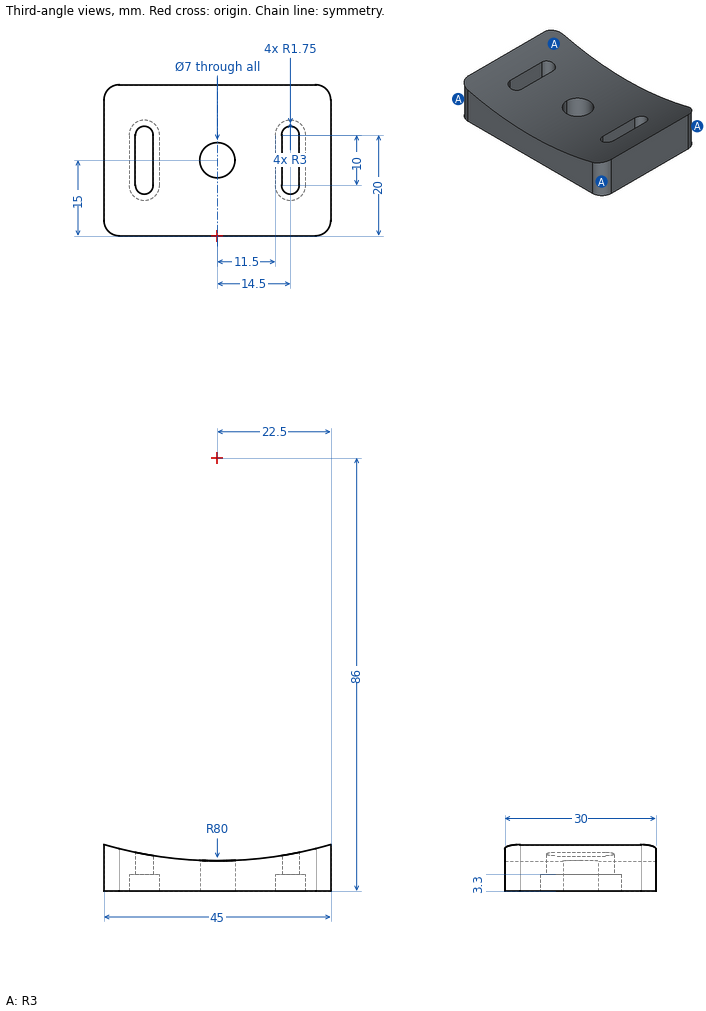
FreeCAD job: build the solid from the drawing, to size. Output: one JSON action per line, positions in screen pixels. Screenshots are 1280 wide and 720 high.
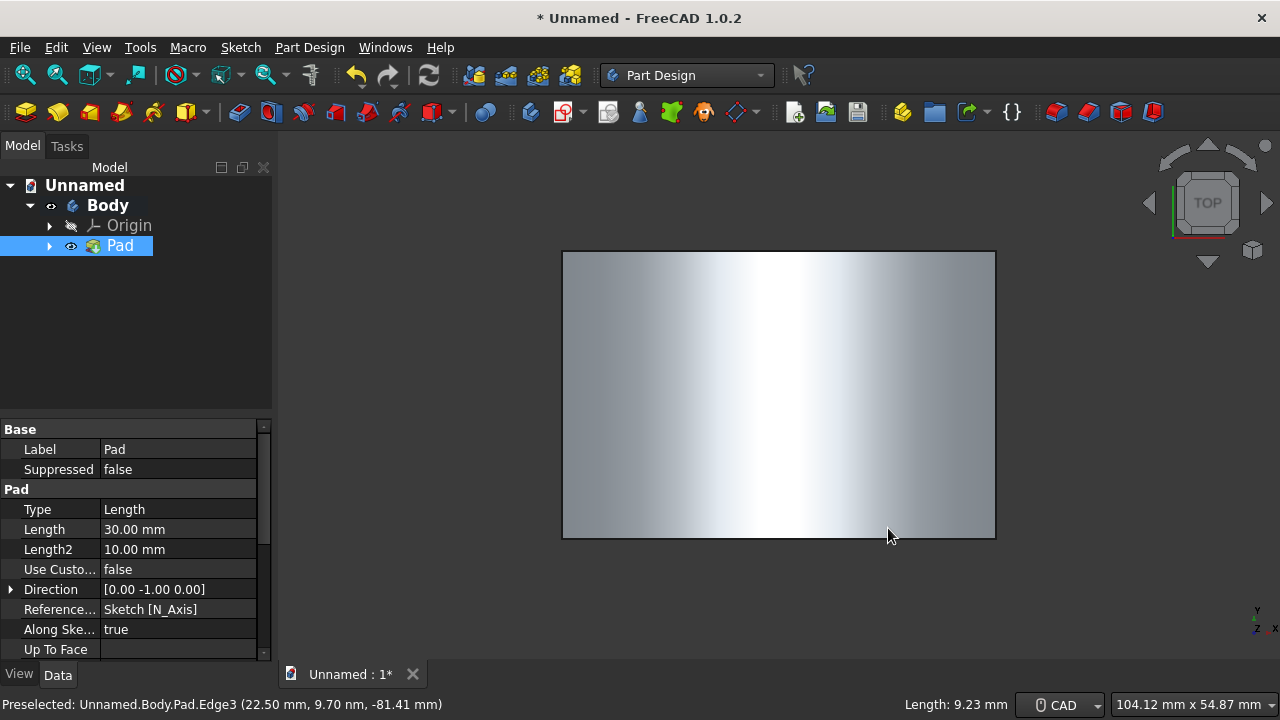
{"action": "key", "text": "1"}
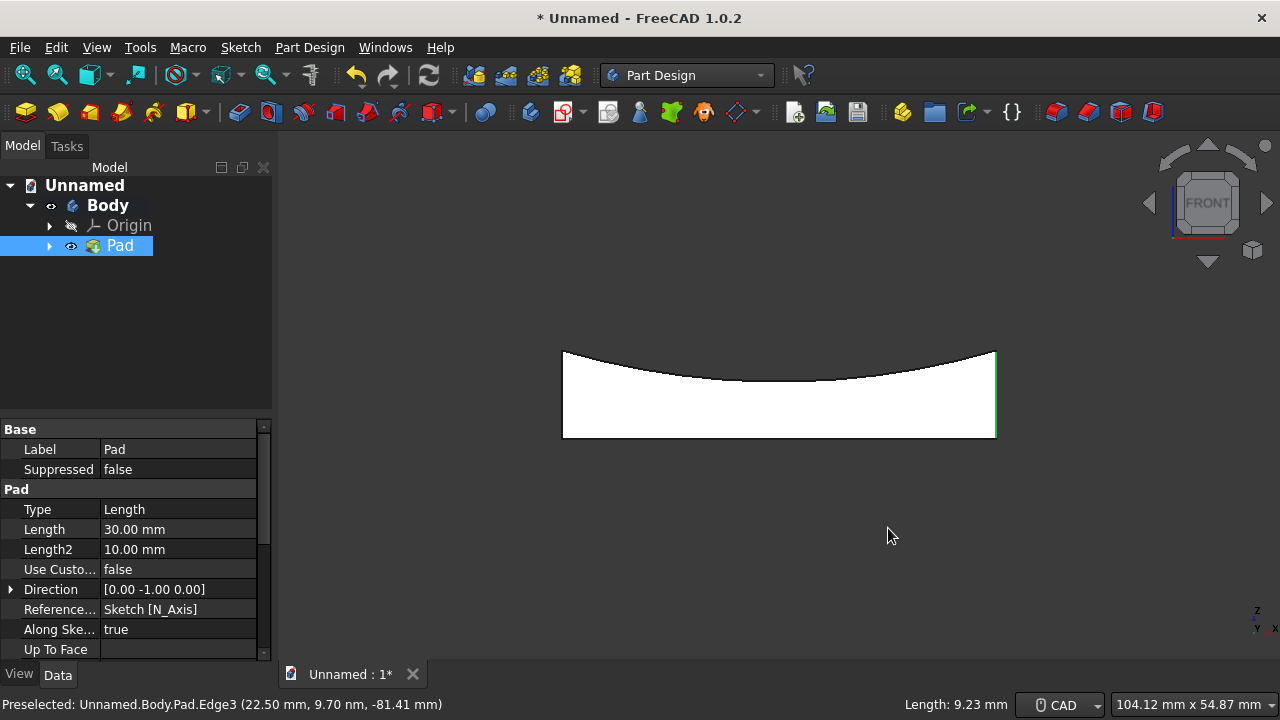
{"action": "left_click", "coordinate": [26, 76]}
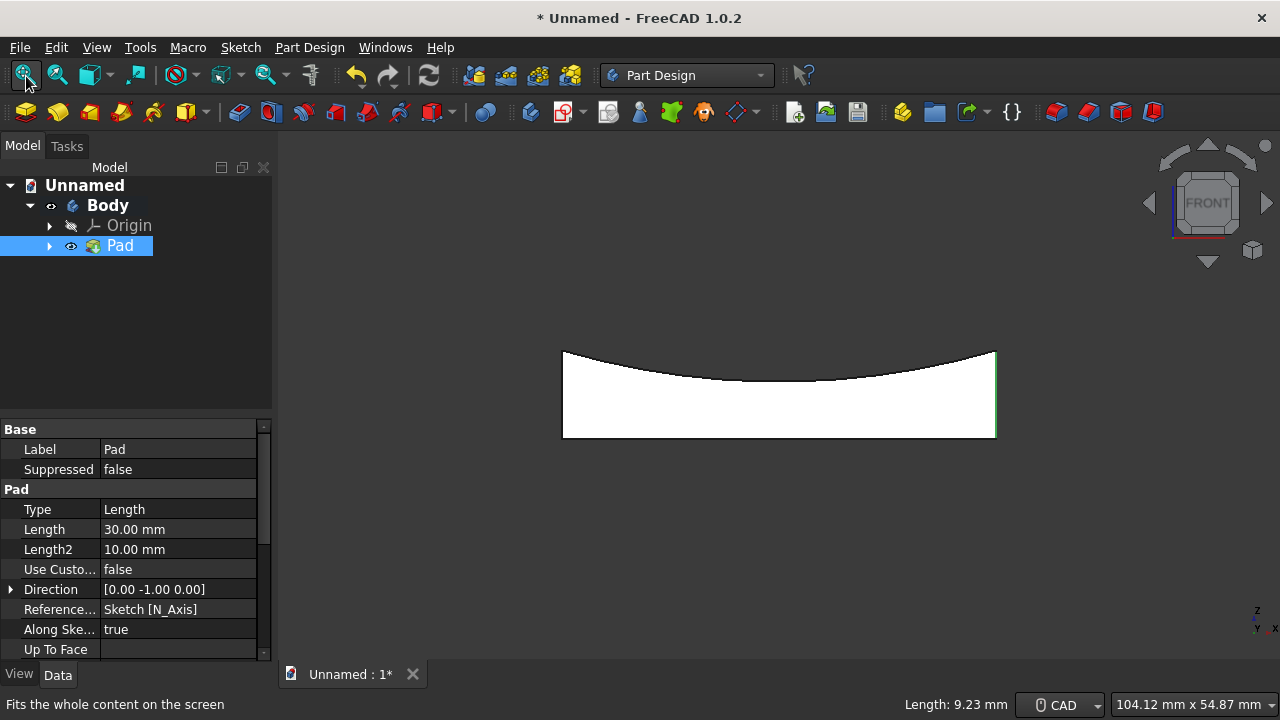
{"action": "left_click", "coordinate": [562, 428], "text": "ctrl"}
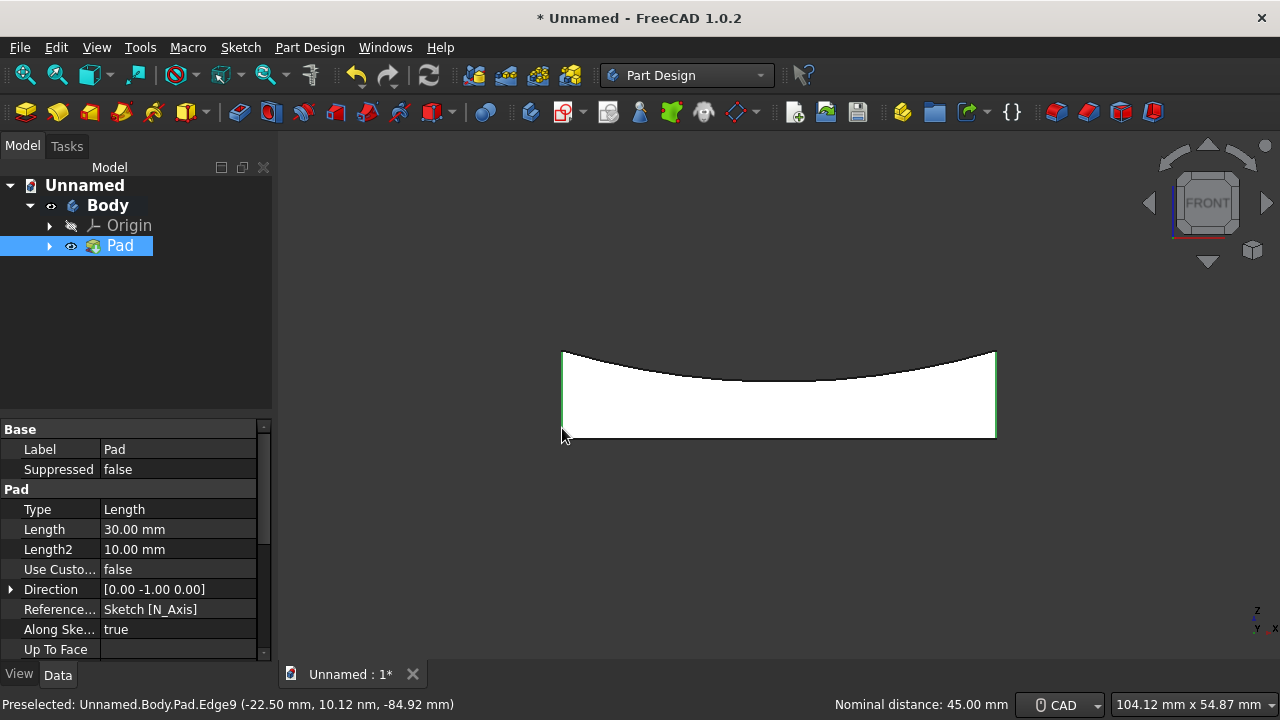
{"action": "key", "text": "3"}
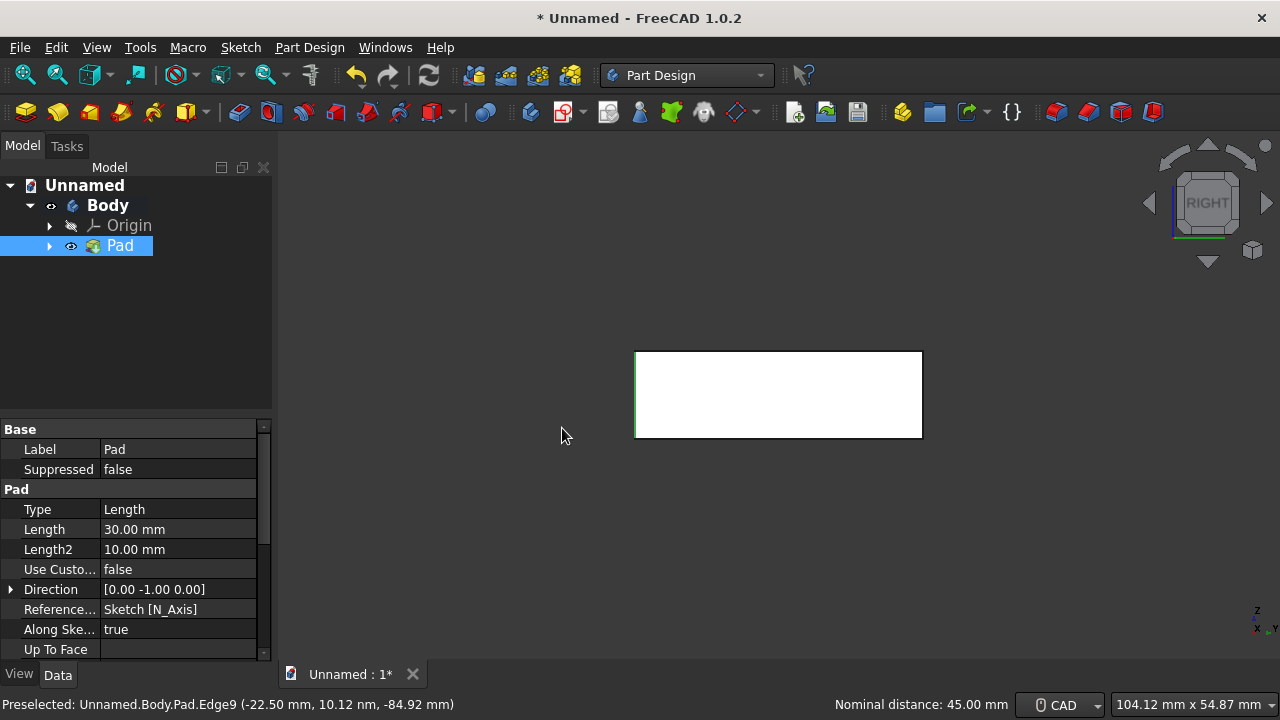
{"action": "key", "text": "v f"}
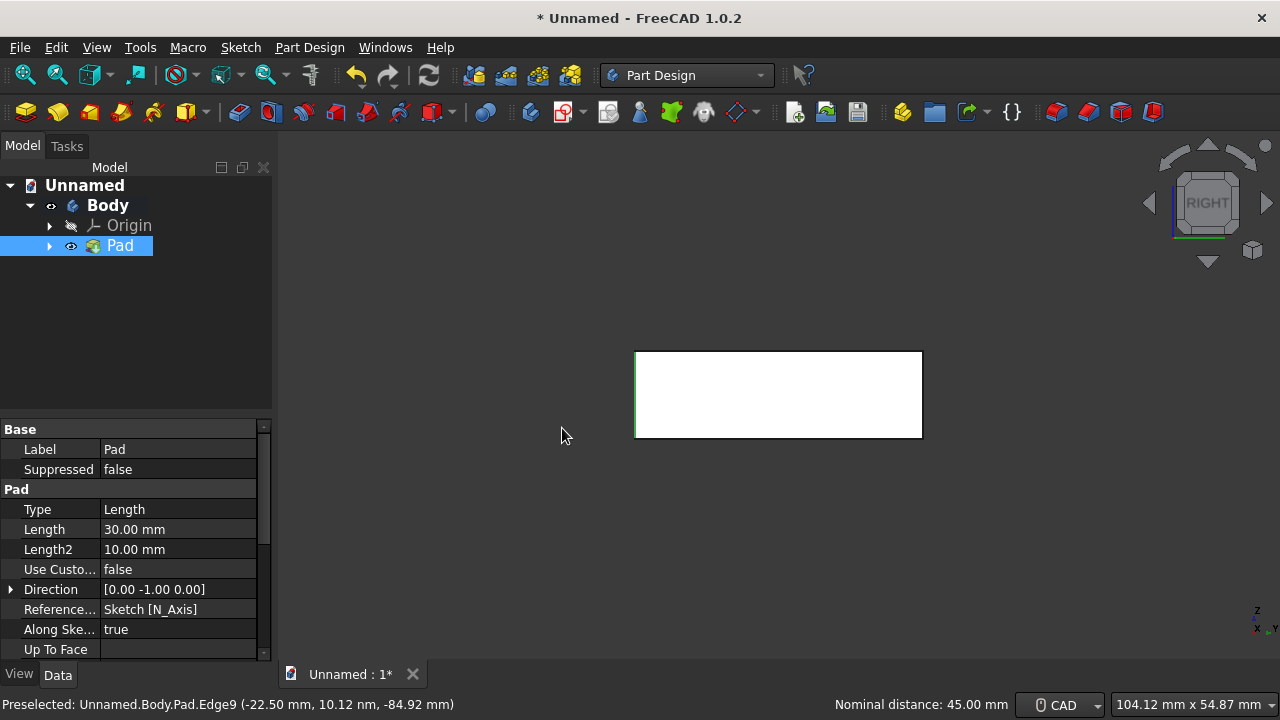
{"action": "left_click", "coordinate": [923, 394], "text": "ctrl"}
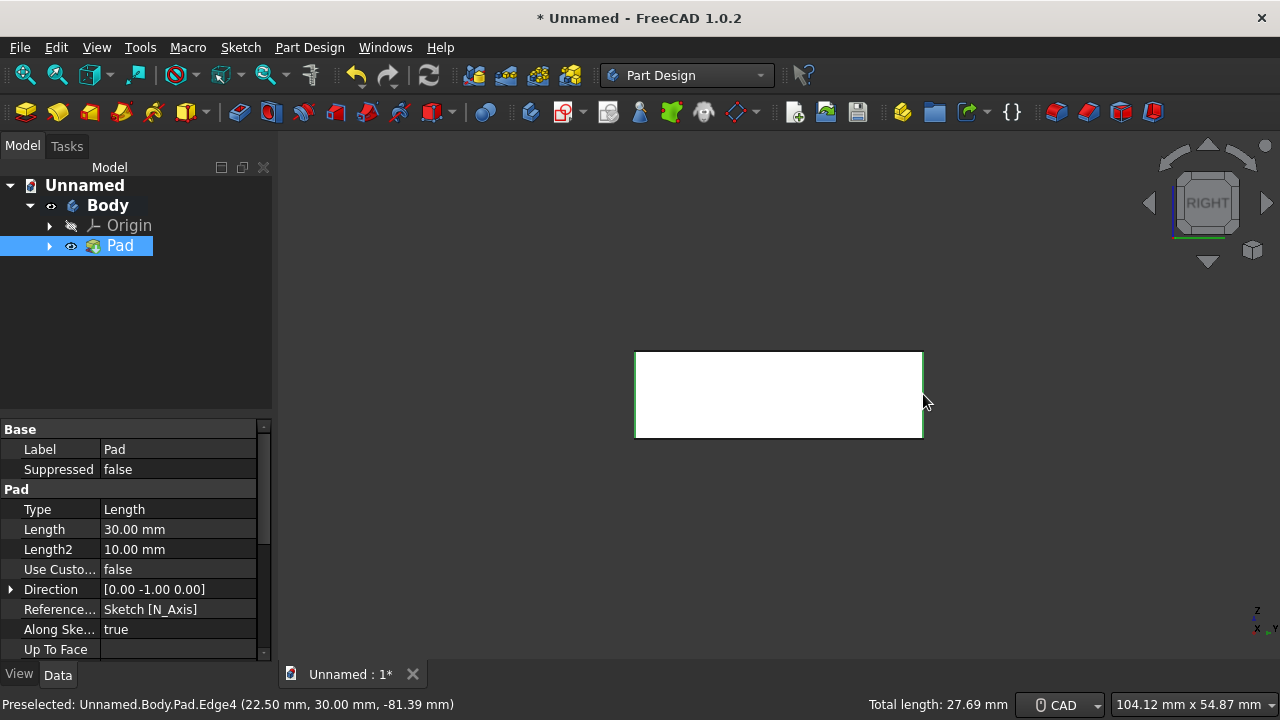
{"action": "key", "text": "5"}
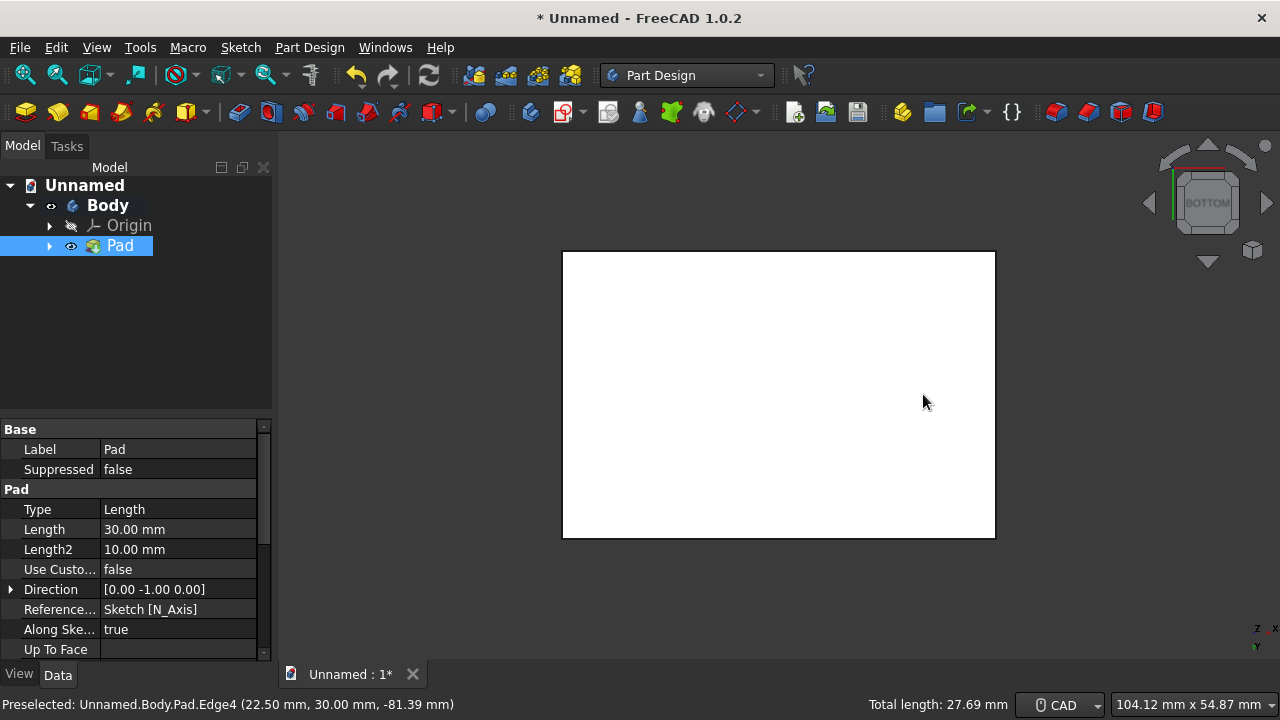
{"action": "key", "text": "4"}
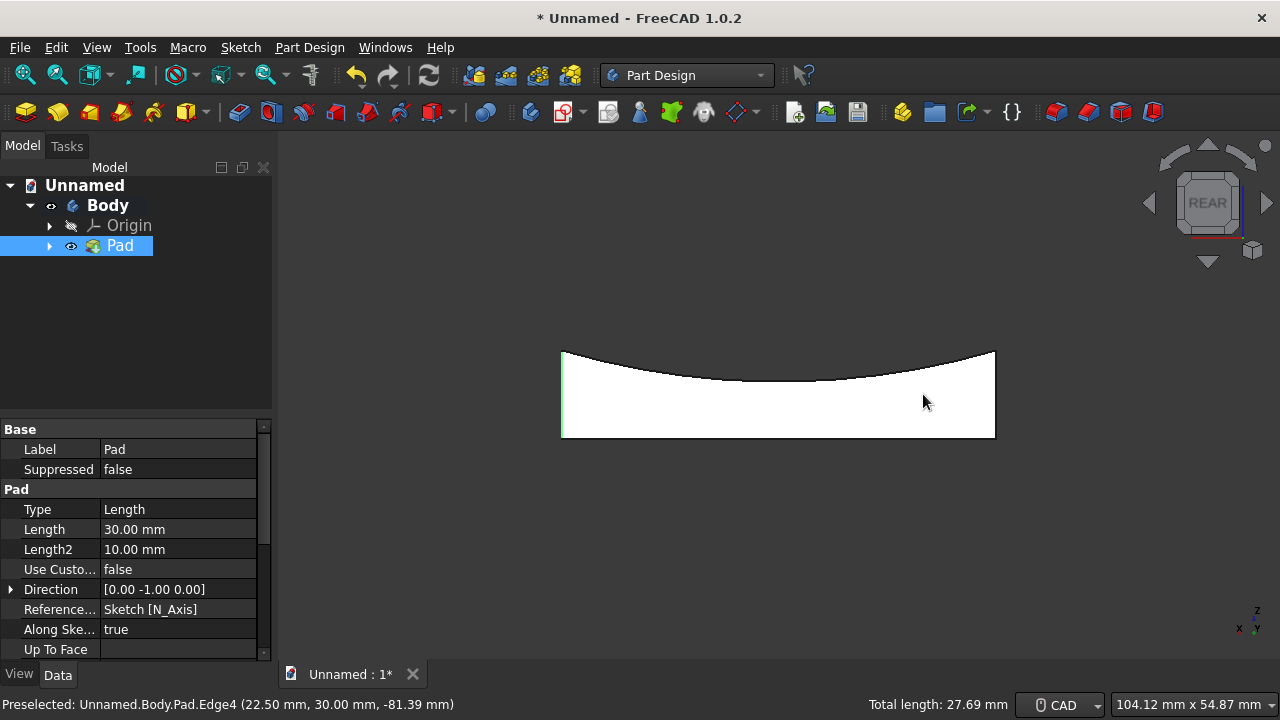
{"action": "left_click", "coordinate": [26, 76]}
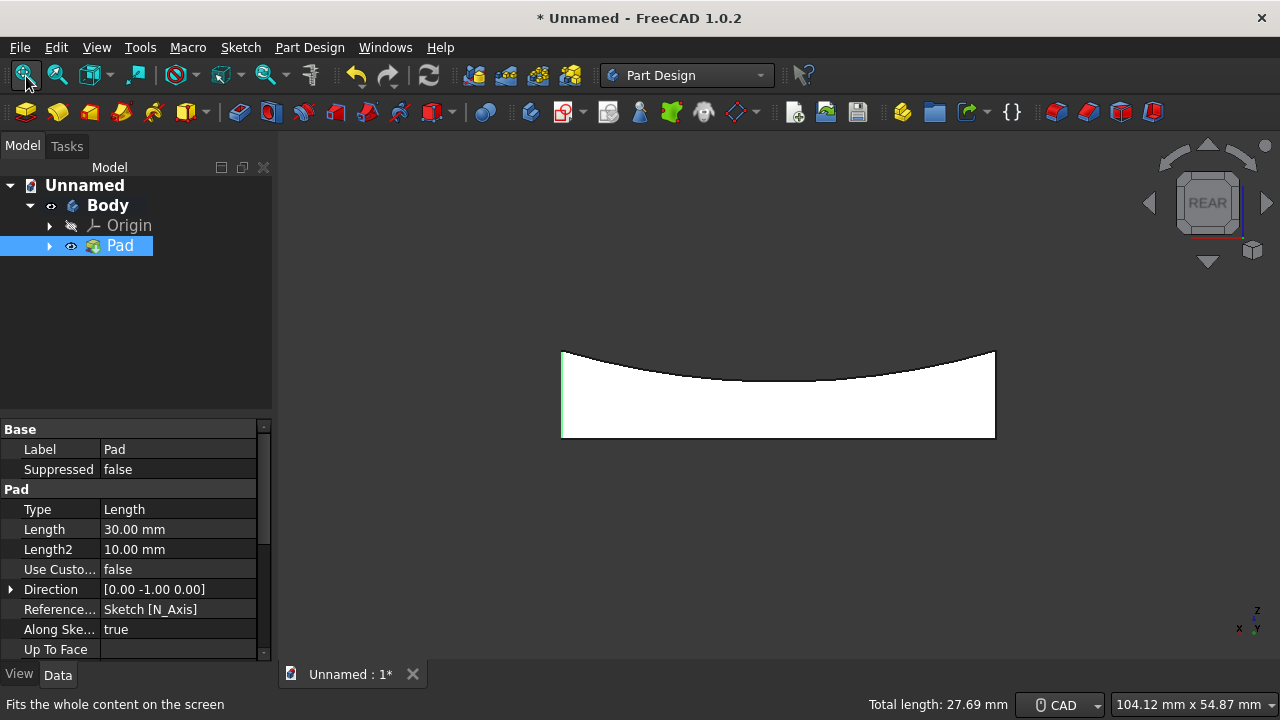
{"action": "left_click", "coordinate": [996, 394], "text": "ctrl"}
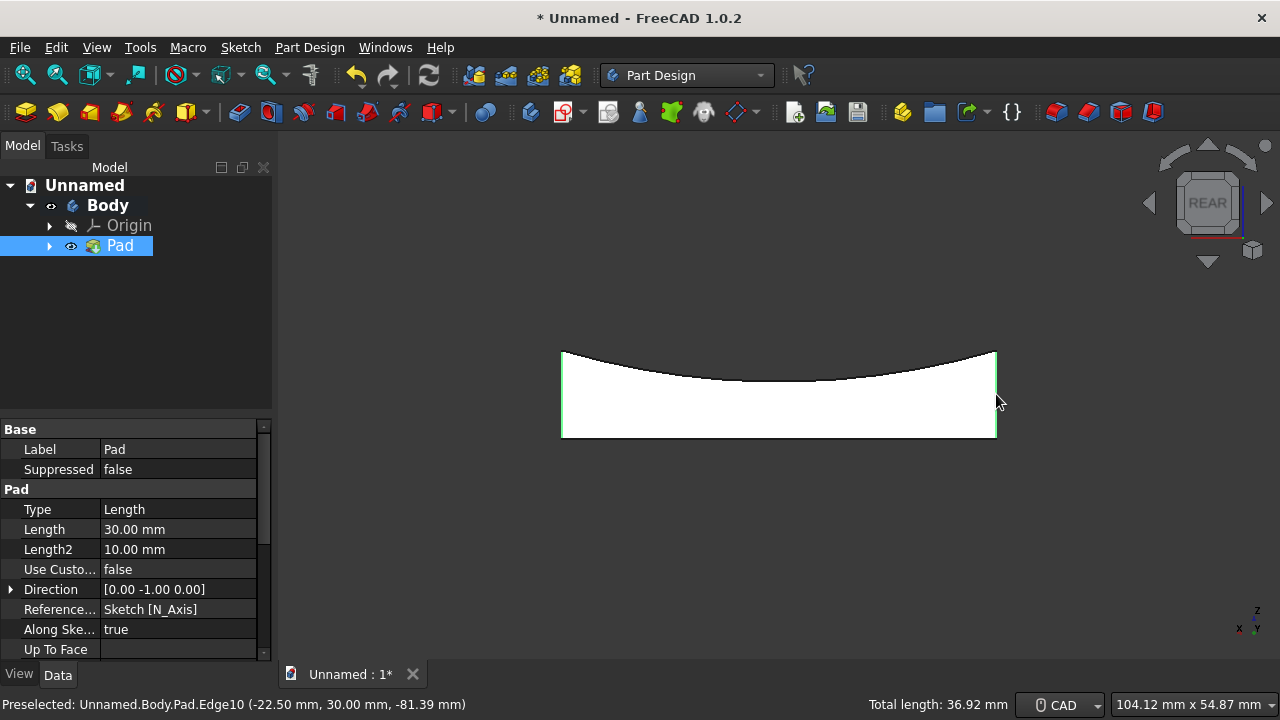
{"action": "left_click", "coordinate": [1058, 112]}